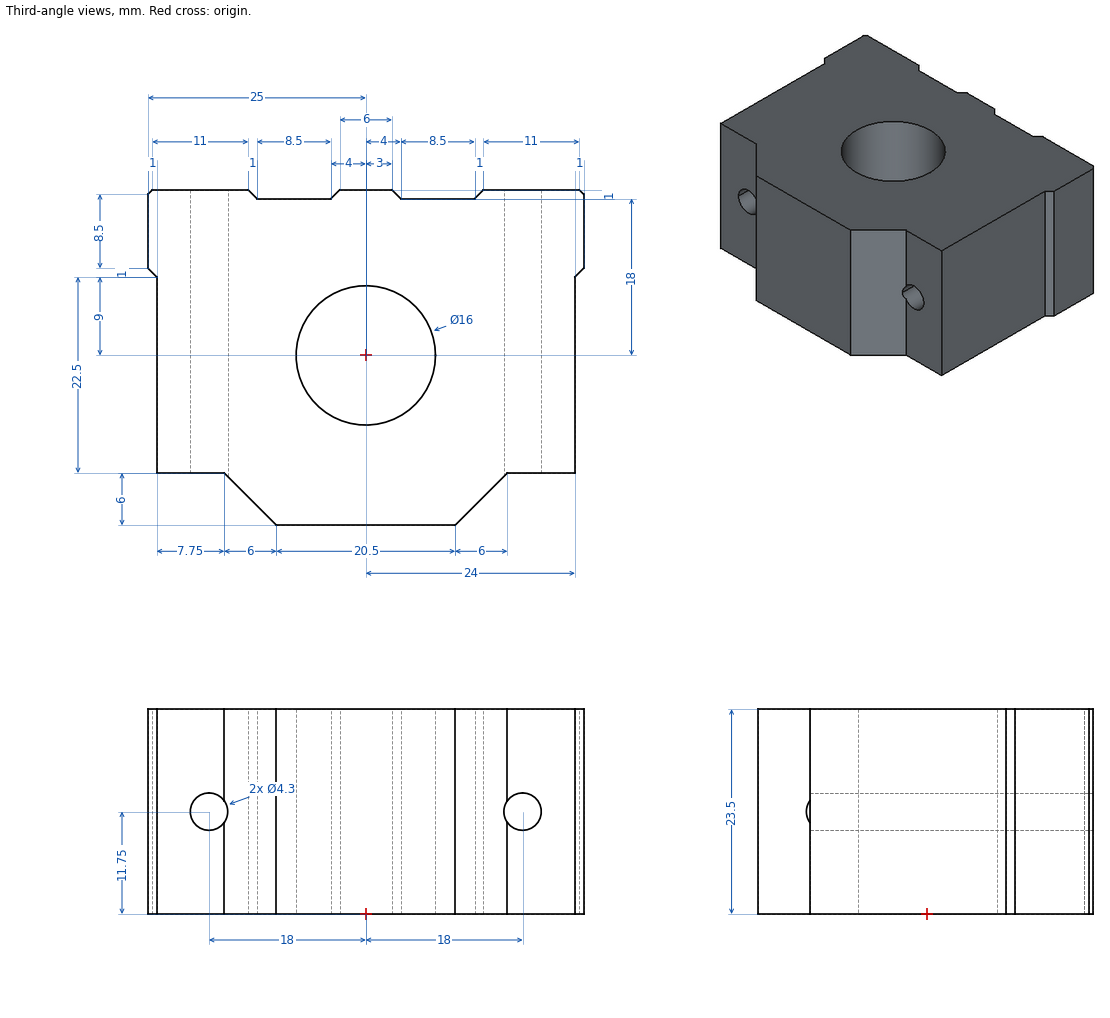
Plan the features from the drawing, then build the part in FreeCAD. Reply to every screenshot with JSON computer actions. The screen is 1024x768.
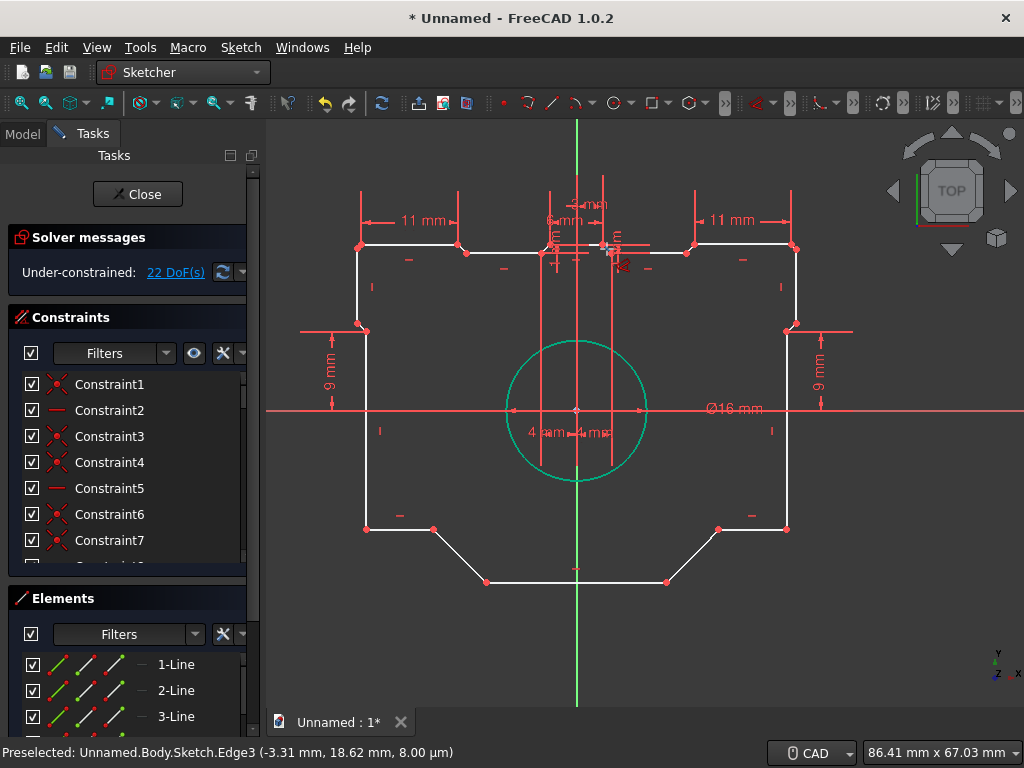
{"action": "scroll", "coordinate": [464, 251], "scroll_direction": "up", "scroll_amount": 8}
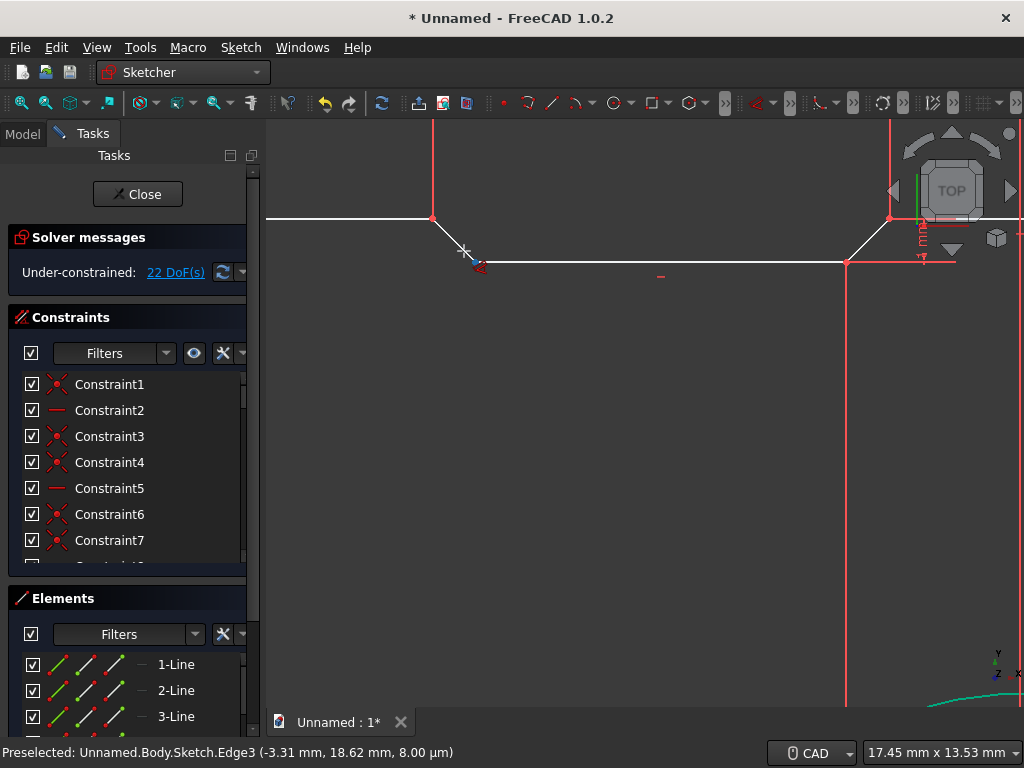
{"action": "left_click", "coordinate": [463, 249]}
{"action": "left_click", "coordinate": [454, 185]}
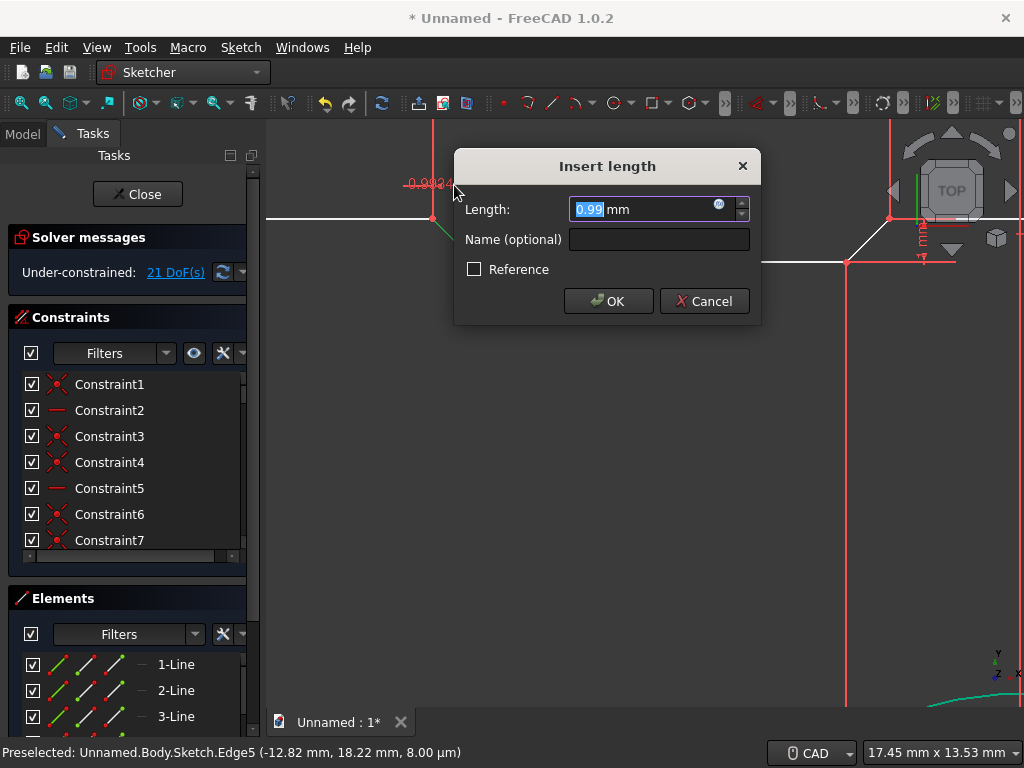
{"action": "type", "text": "1"}
{"action": "key", "text": "Return"}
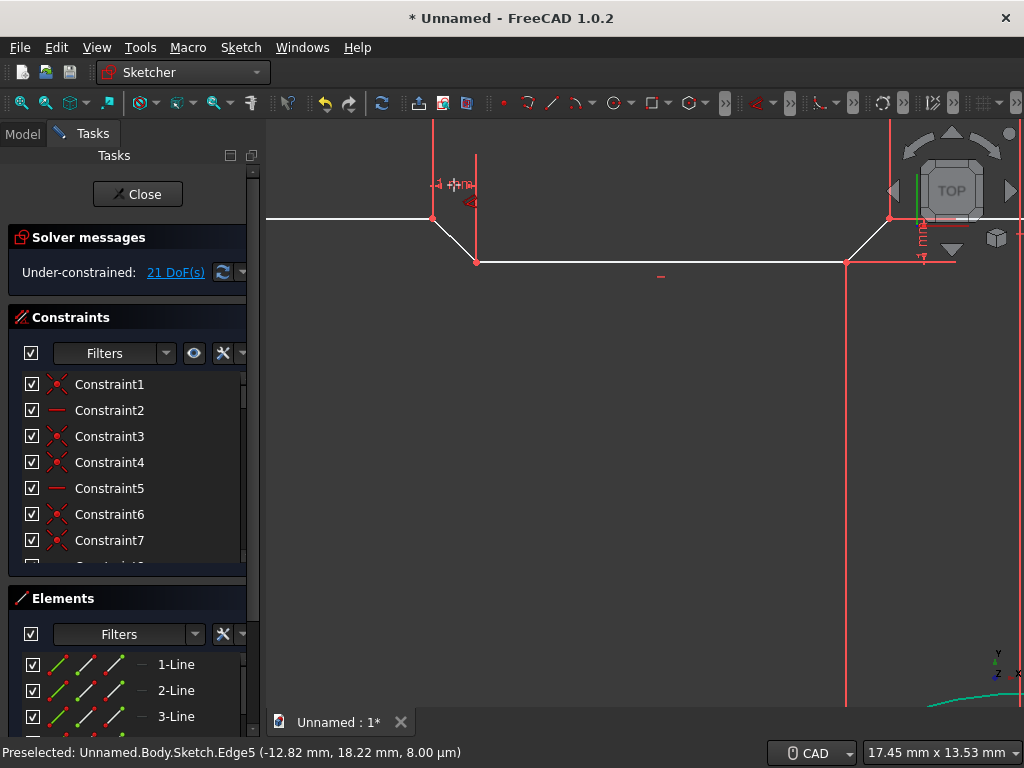
{"action": "left_click", "coordinate": [463, 249]}
{"action": "left_click", "coordinate": [399, 240]}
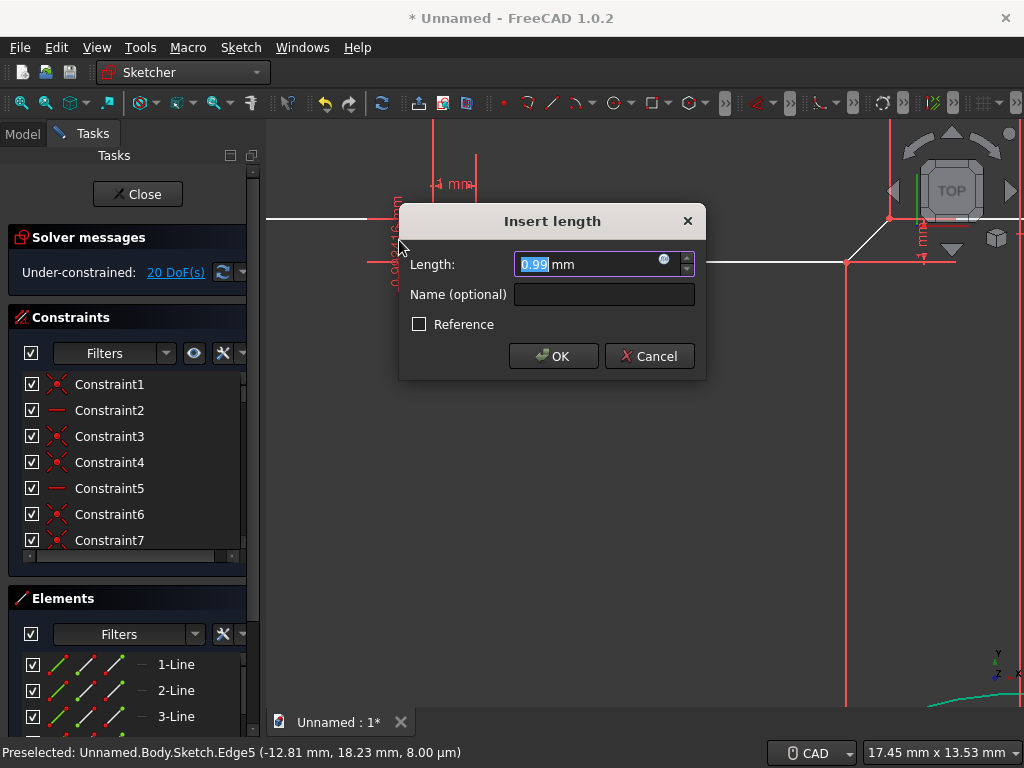
{"action": "type", "text": "1"}
{"action": "key", "text": "Return"}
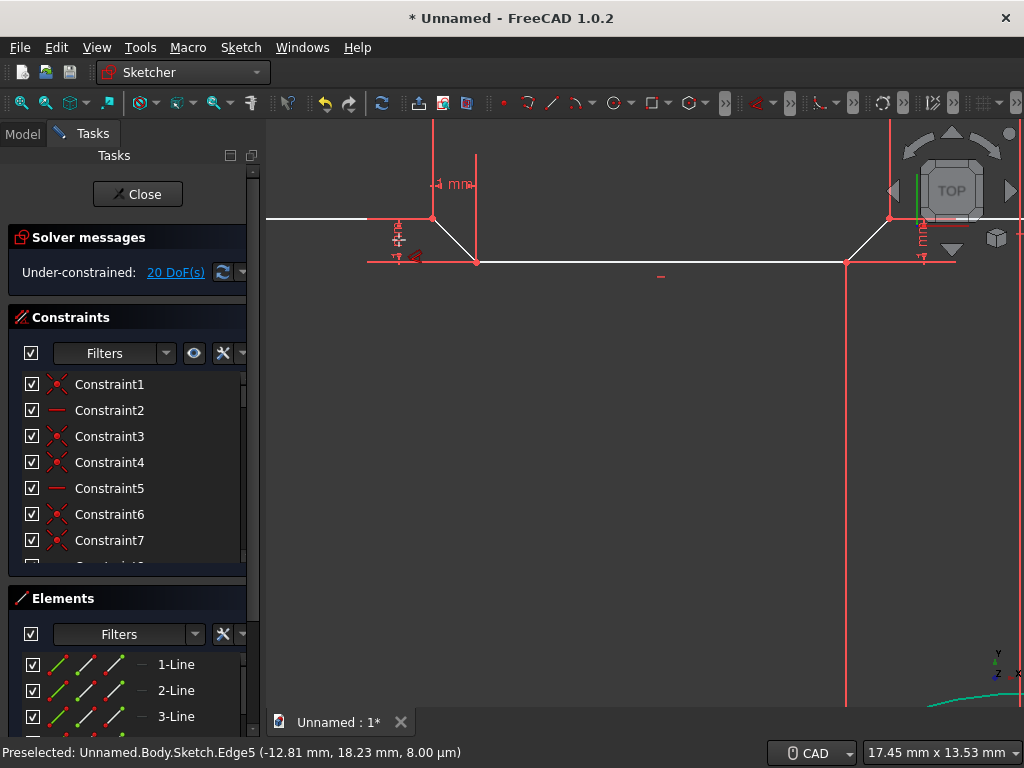
{"action": "scroll", "coordinate": [464, 251], "scroll_direction": "down", "scroll_amount": 8}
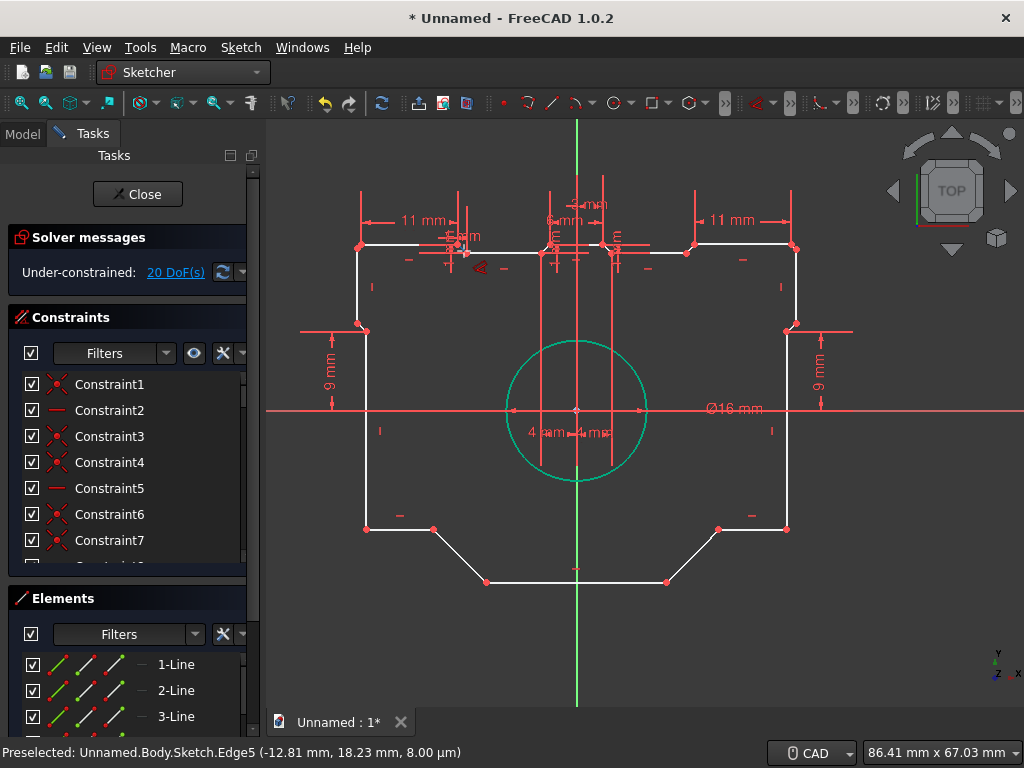
{"action": "scroll", "coordinate": [360, 326], "scroll_direction": "up", "scroll_amount": 8}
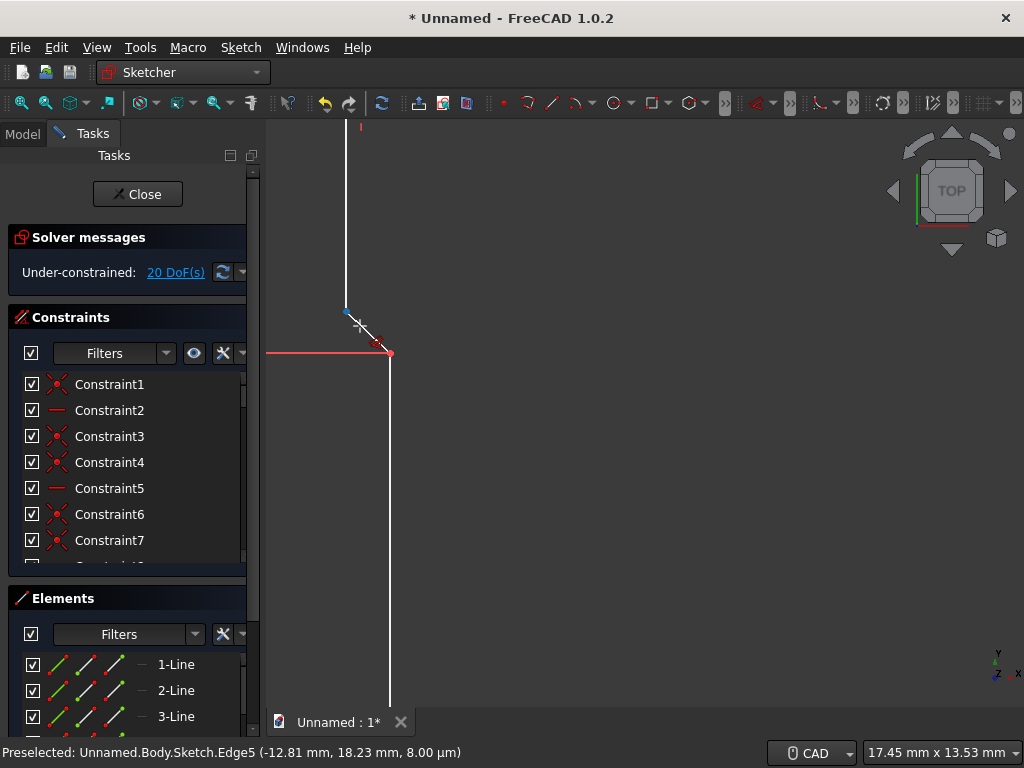
{"action": "left_click", "coordinate": [359, 324]}
{"action": "left_click", "coordinate": [368, 278]}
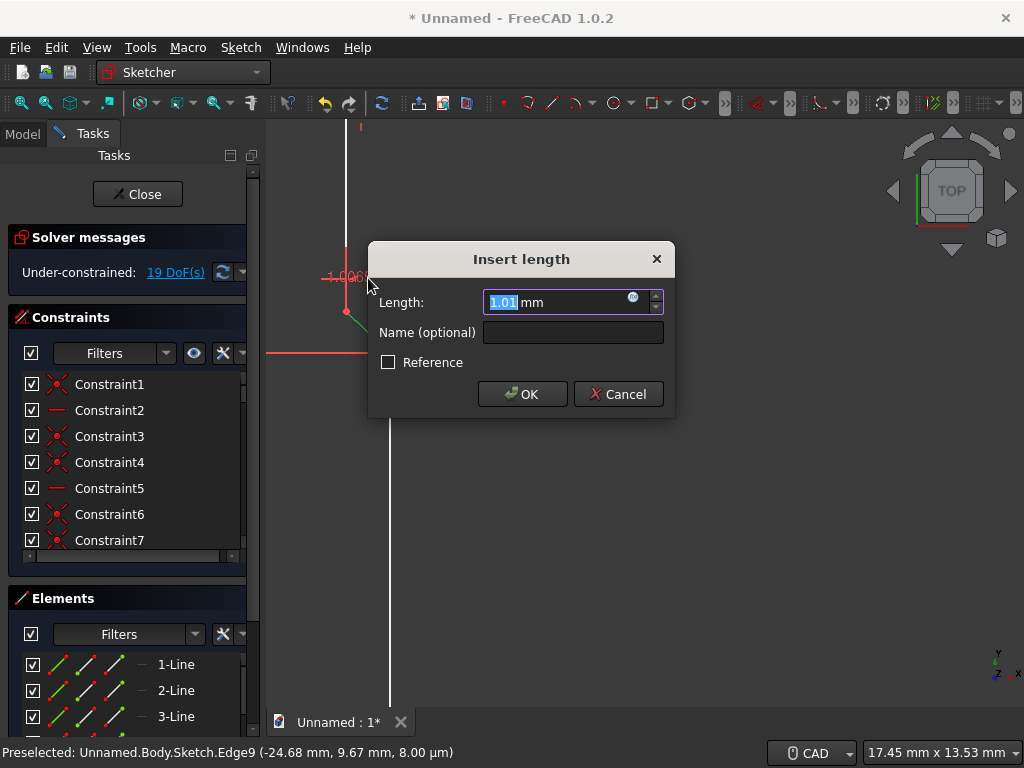
{"action": "type", "text": "1"}
{"action": "key", "text": "Return"}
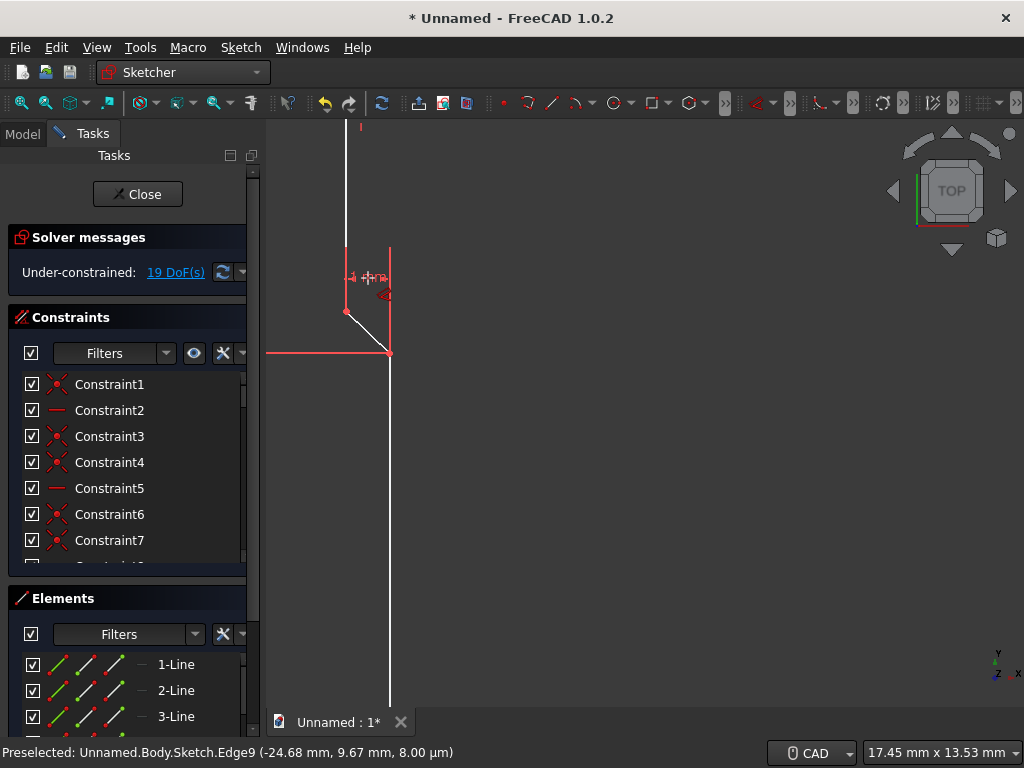
{"action": "left_click", "coordinate": [359, 324]}
{"action": "left_click", "coordinate": [312, 333]}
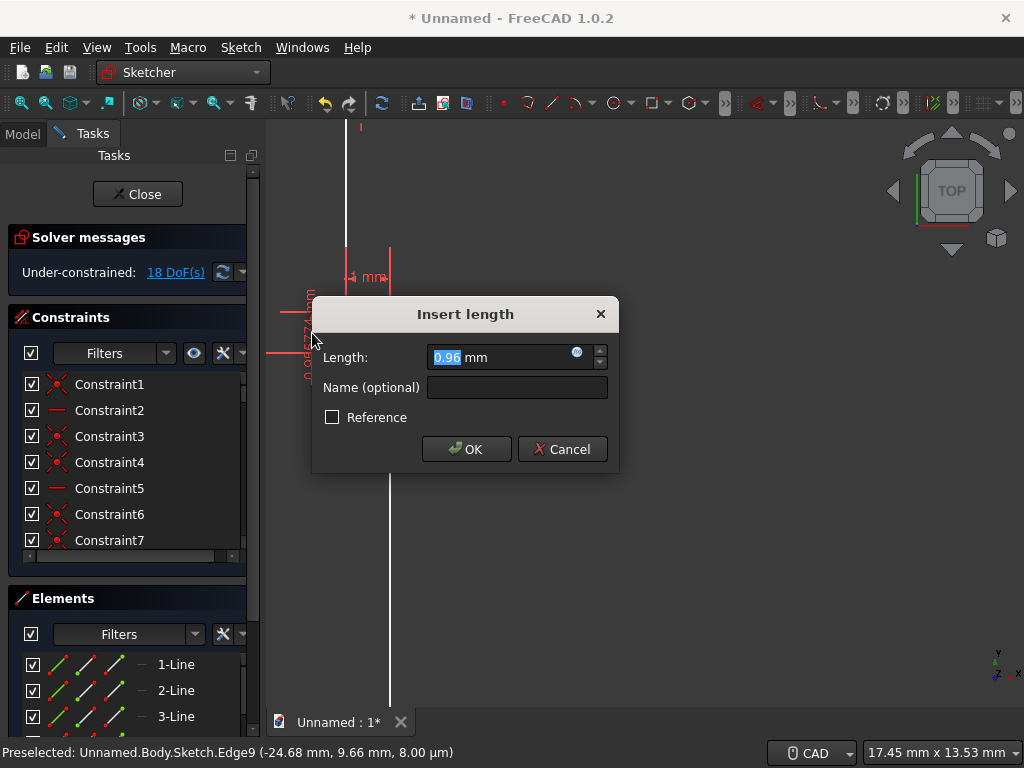
{"action": "type", "text": "1"}
{"action": "key", "text": "Return"}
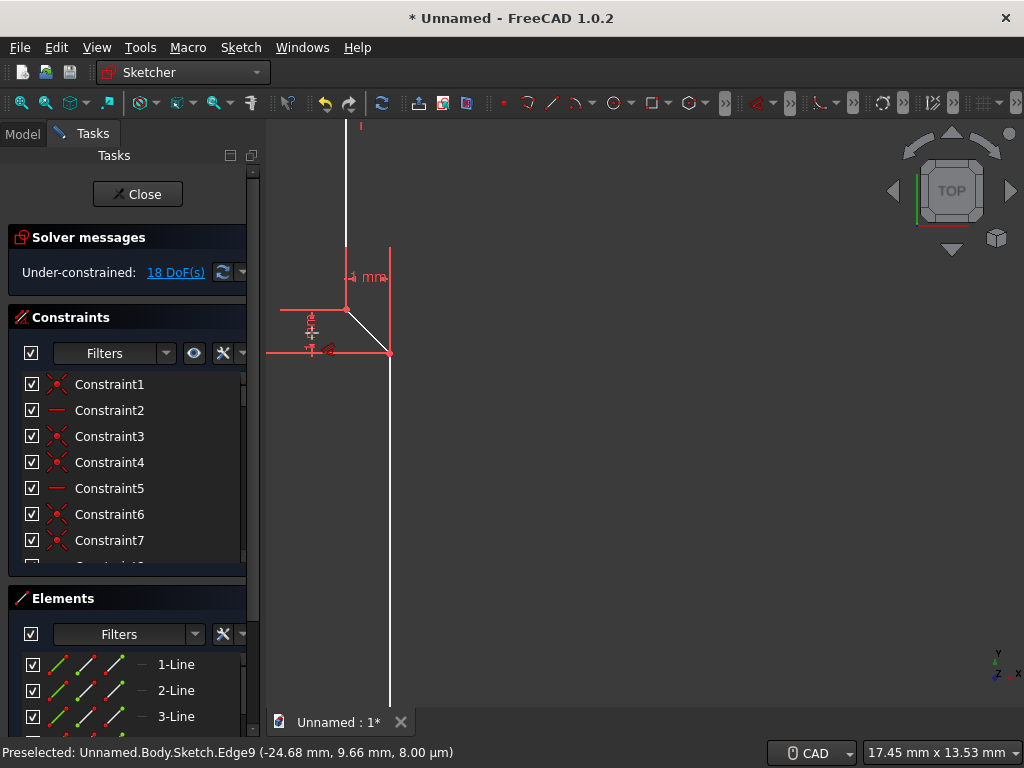
{"action": "scroll", "coordinate": [360, 326], "scroll_direction": "down", "scroll_amount": 8}